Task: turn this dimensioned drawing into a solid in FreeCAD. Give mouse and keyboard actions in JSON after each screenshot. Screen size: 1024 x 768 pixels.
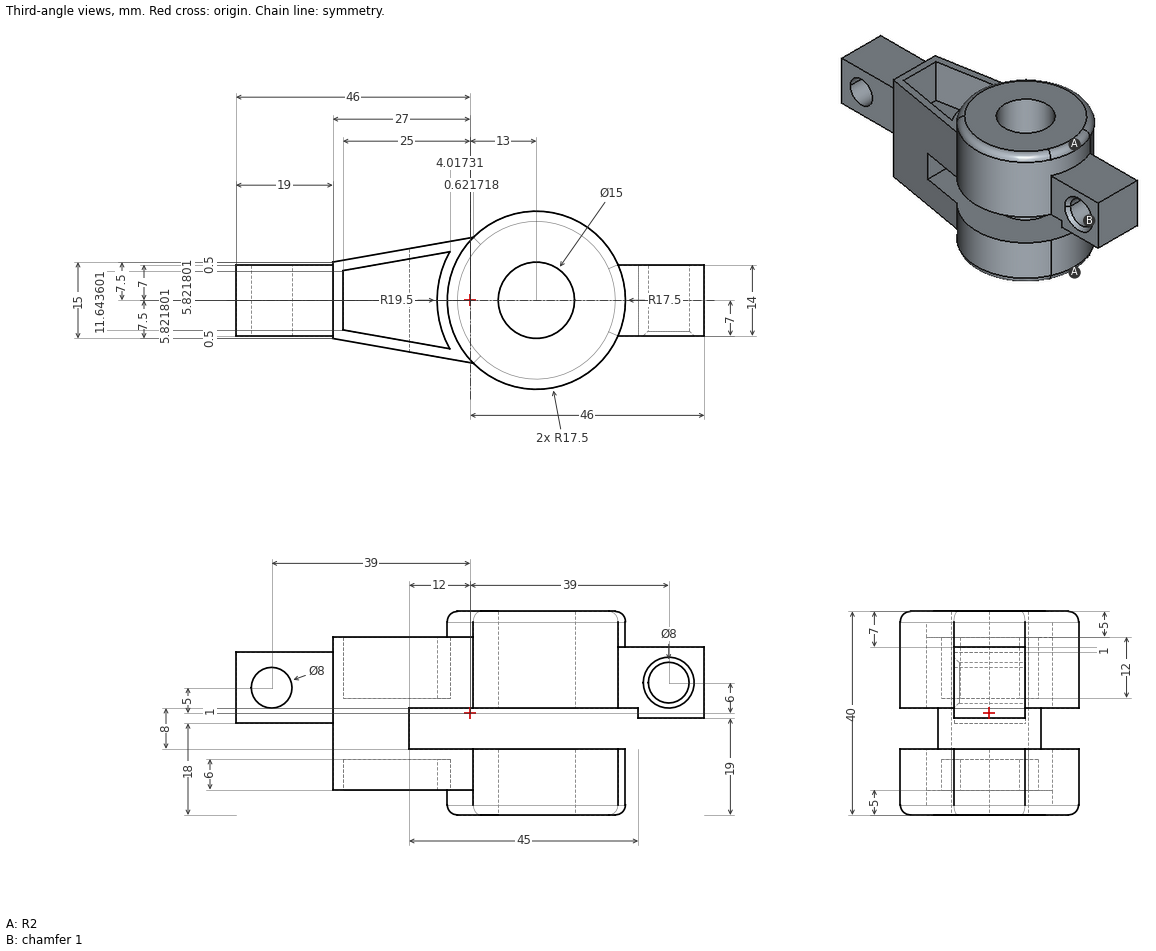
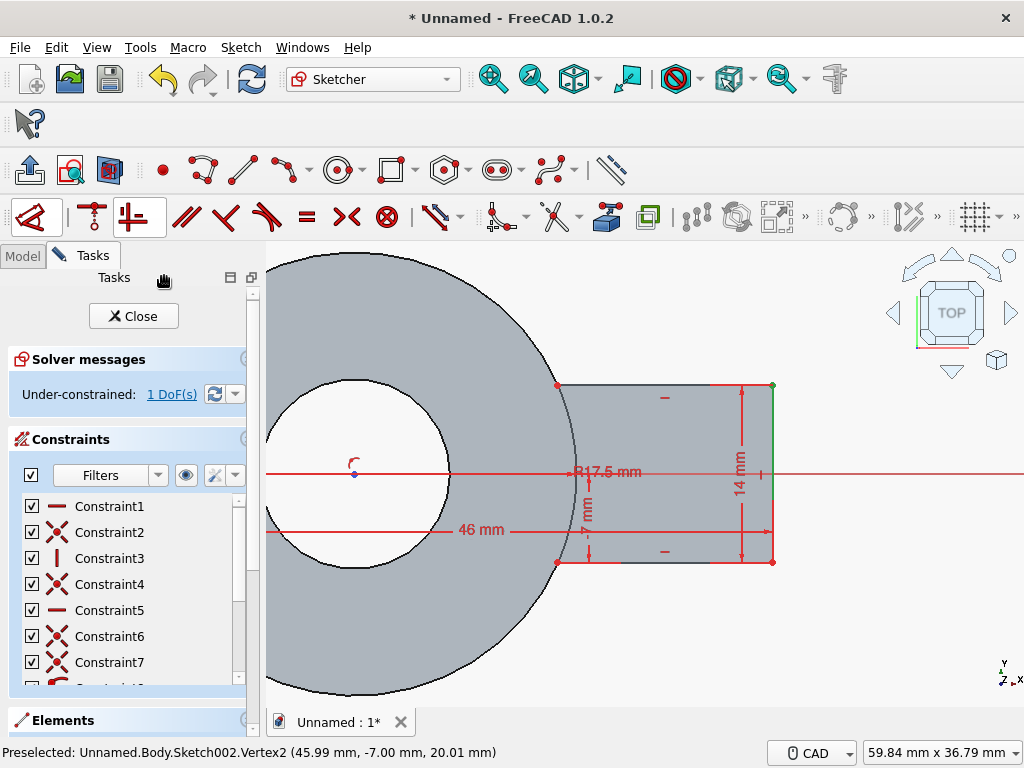
{"action": "left_click", "coordinate": [355, 474]}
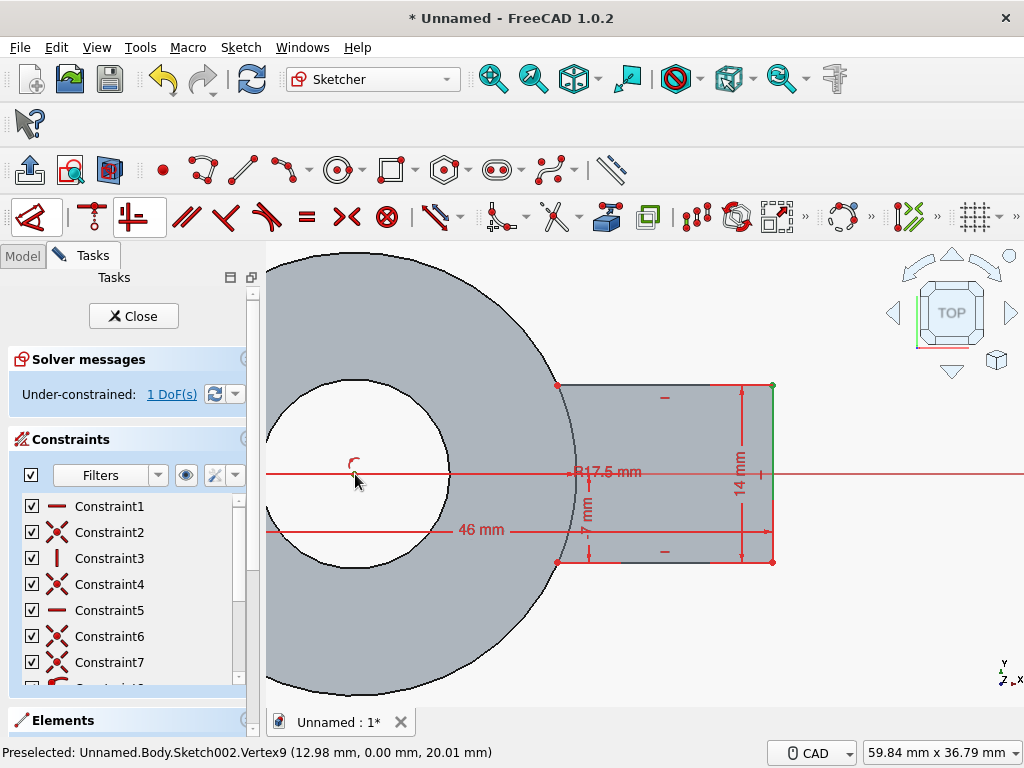
{"action": "key", "text": "l"}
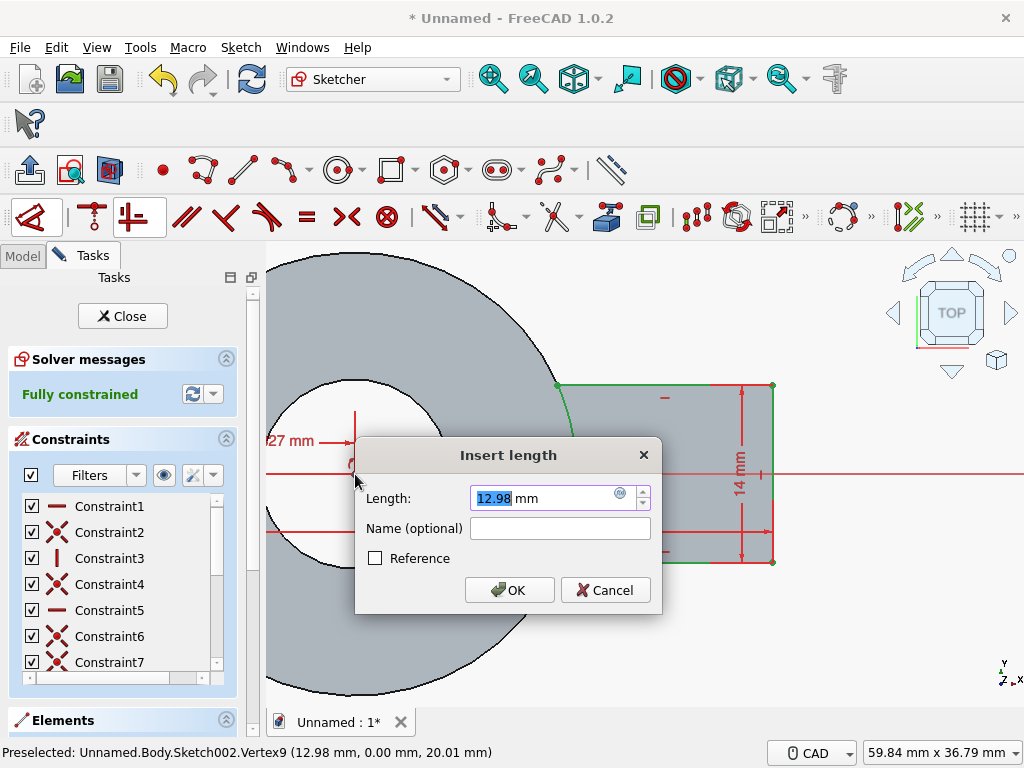
{"action": "type", "text": "13"}
{"action": "key", "text": "Return"}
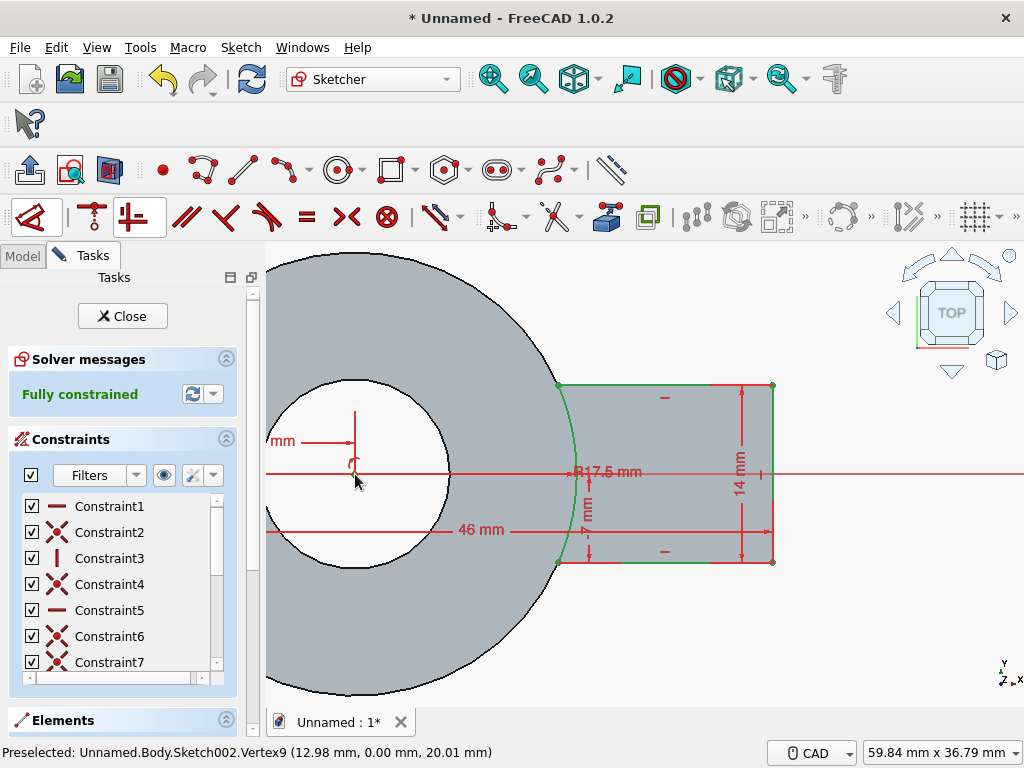
{"action": "left_click", "coordinate": [123, 316]}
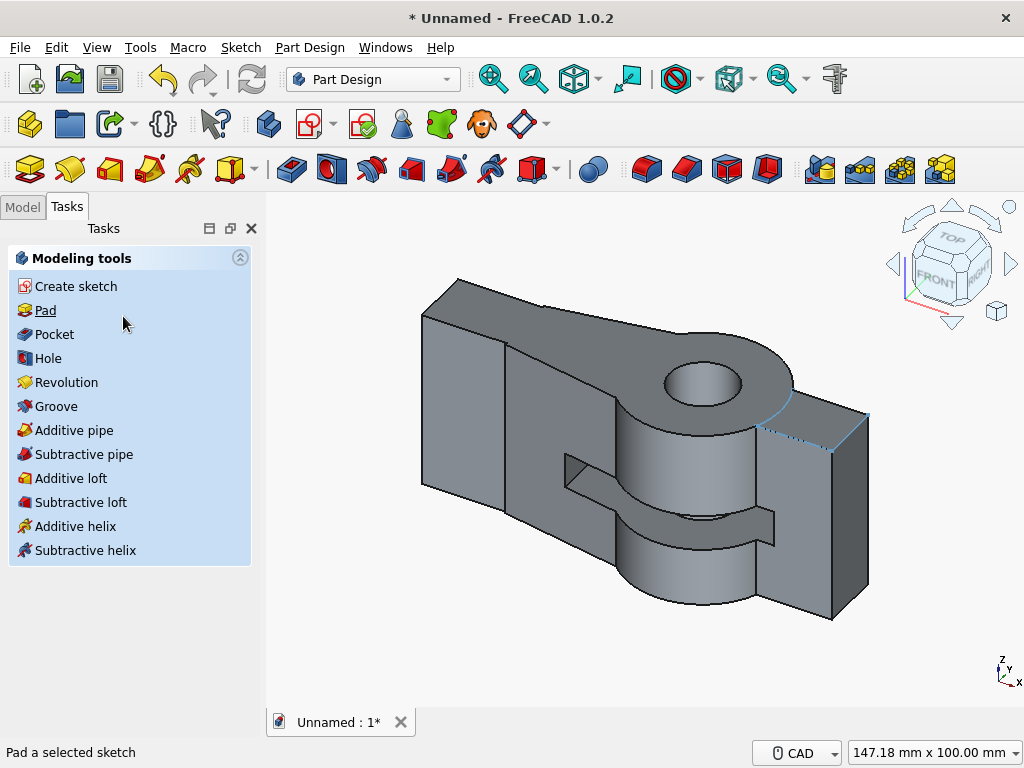
{"action": "left_click", "coordinate": [292, 170]}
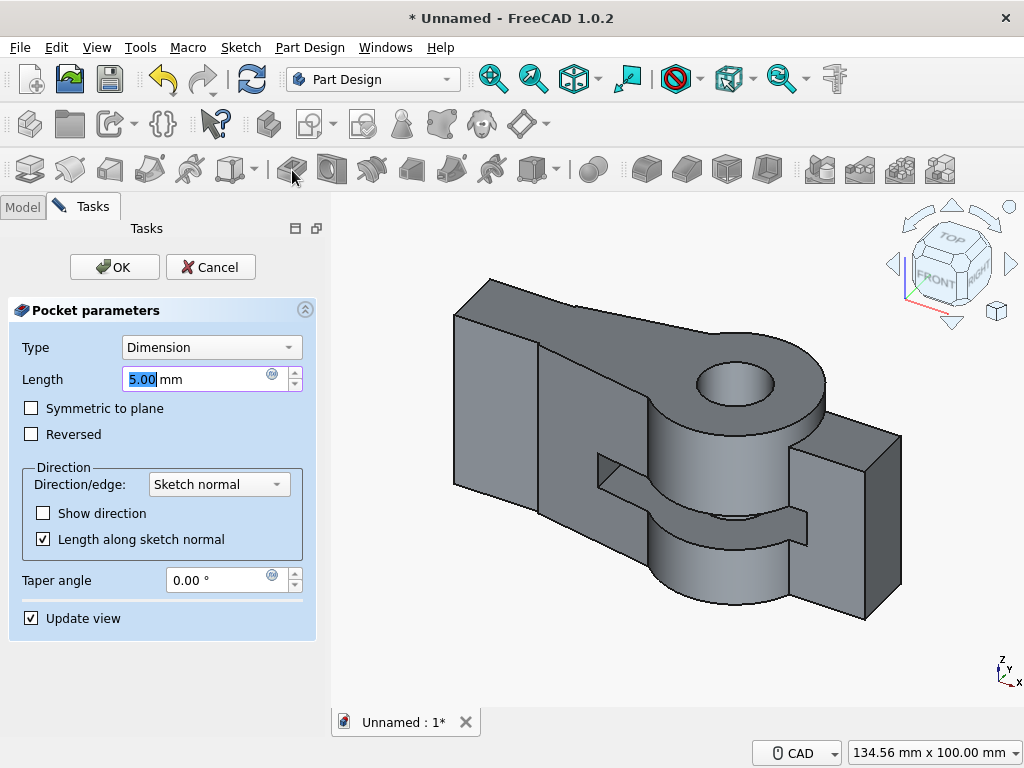
{"action": "type", "text": "7"}
{"action": "key", "text": "Tab"}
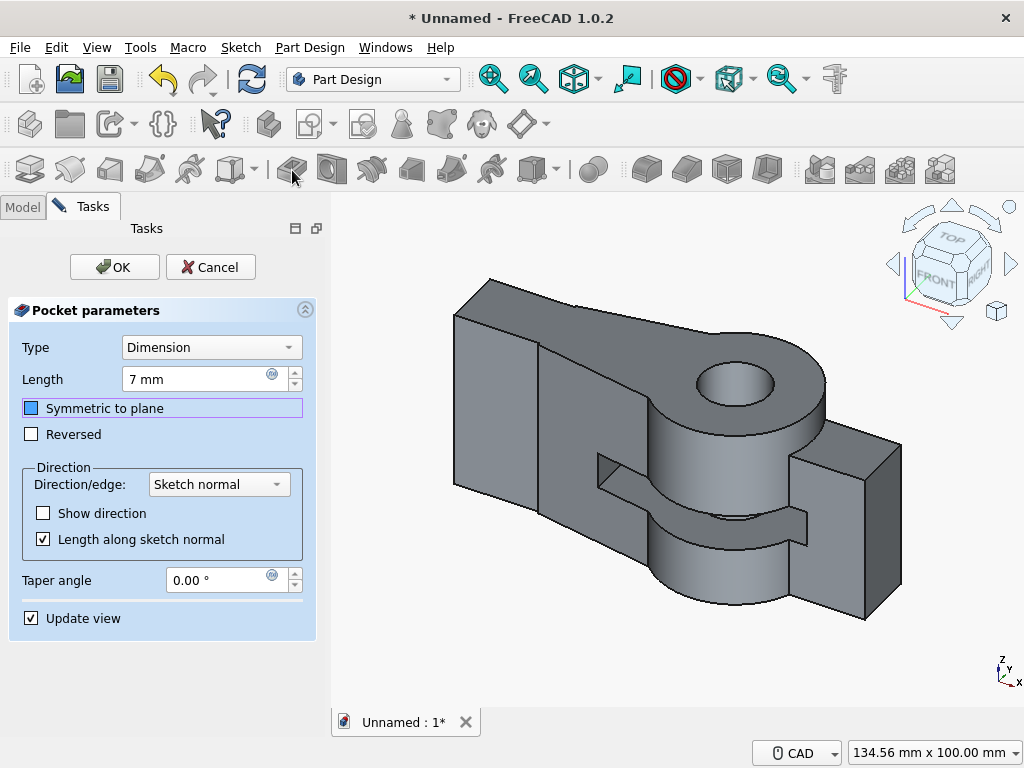
{"action": "left_click", "coordinate": [115, 267]}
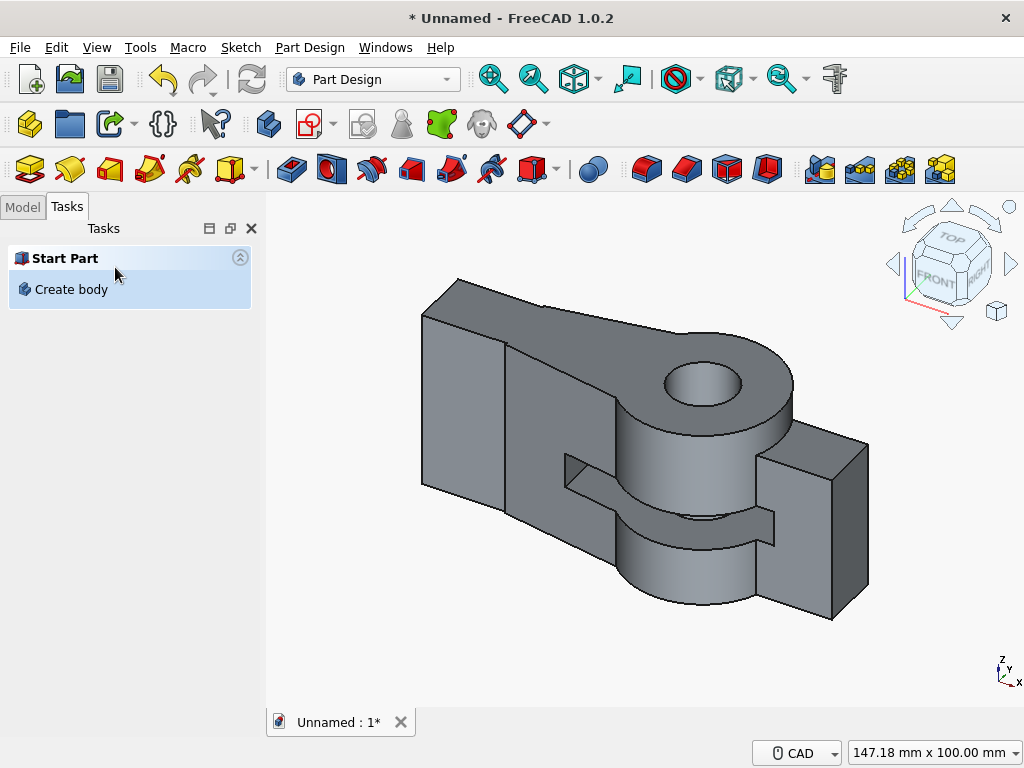
{"action": "left_click", "coordinate": [610, 353]}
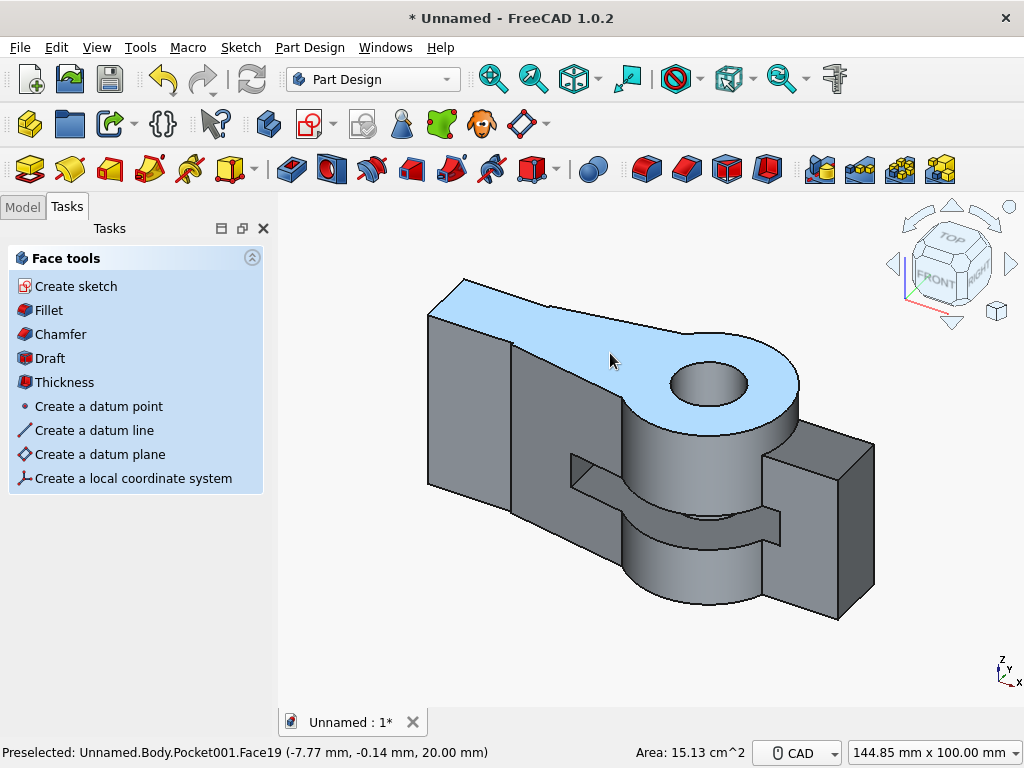
{"action": "left_click", "coordinate": [310, 124]}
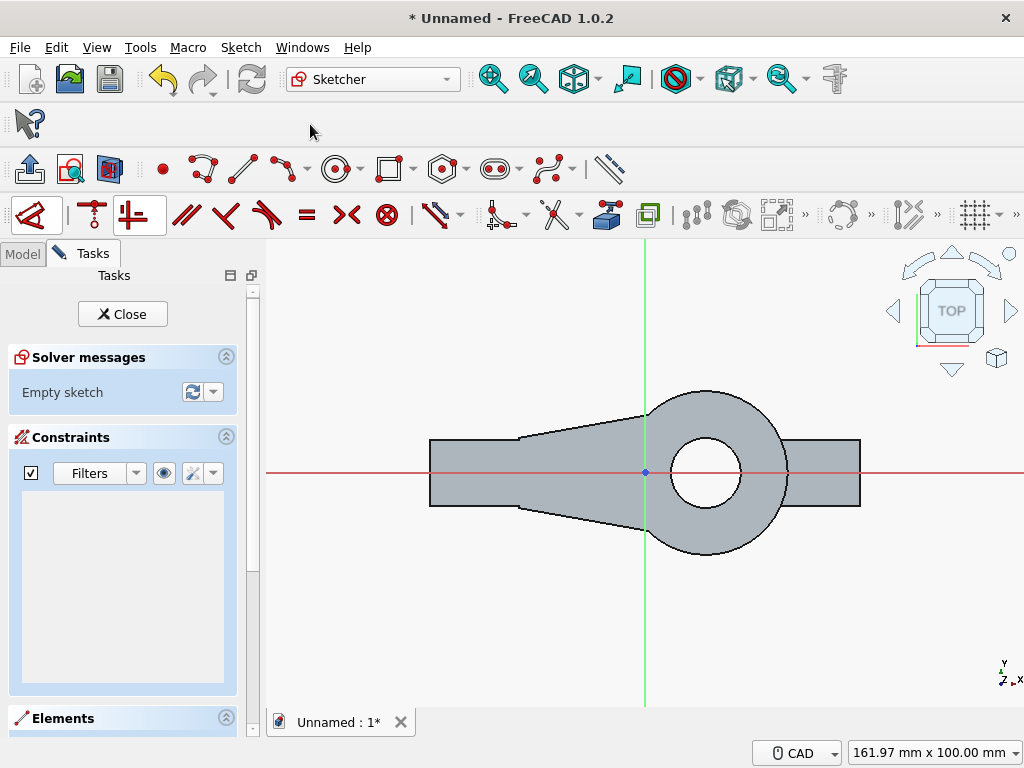
{"action": "scroll", "coordinate": [490, 473], "scroll_direction": "up", "scroll_amount": 3}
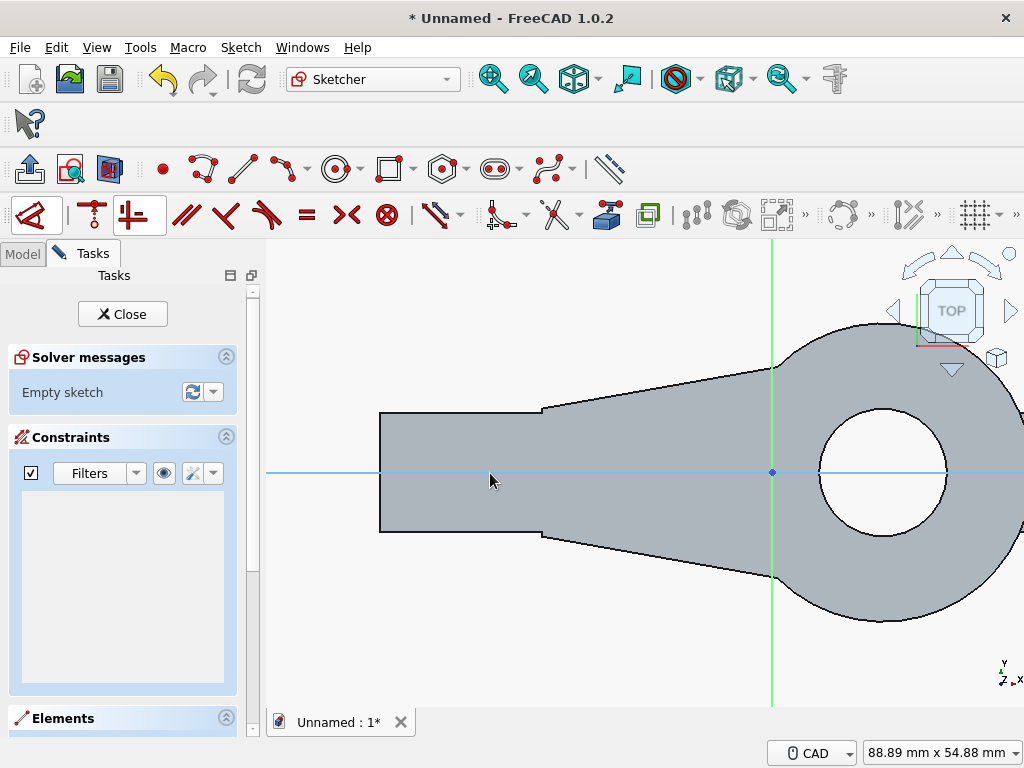
{"action": "left_click", "coordinate": [390, 170]}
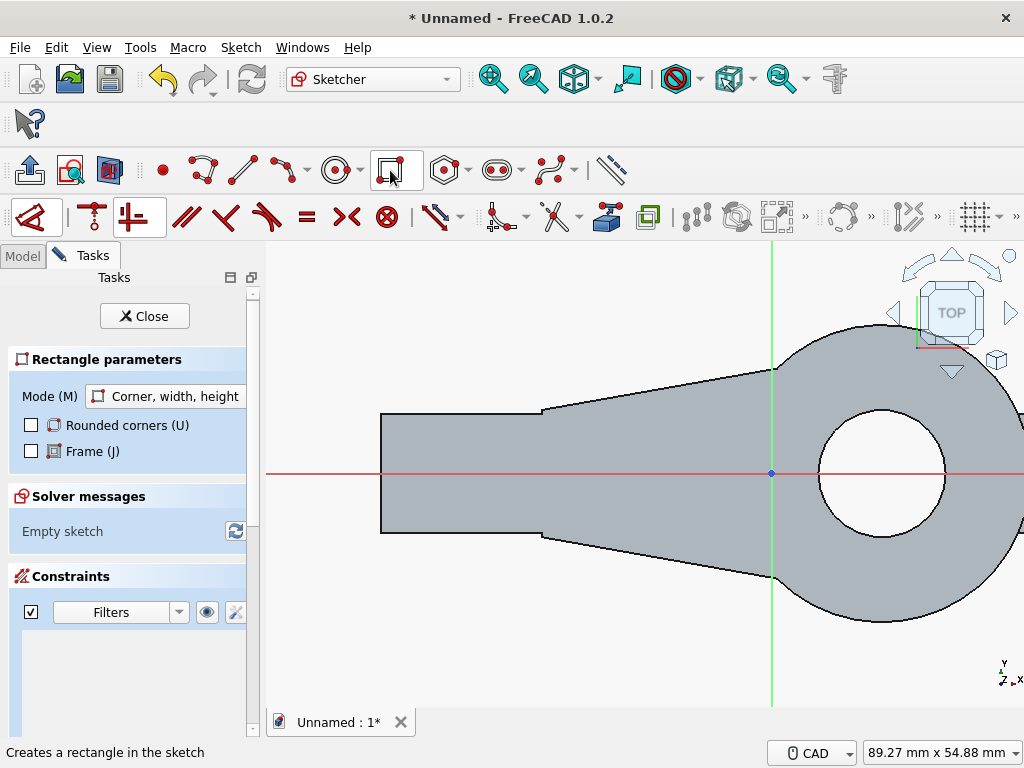
{"action": "left_click", "coordinate": [381, 414]}
{"action": "left_click", "coordinate": [542, 533]}
{"action": "key", "text": "Escape"}